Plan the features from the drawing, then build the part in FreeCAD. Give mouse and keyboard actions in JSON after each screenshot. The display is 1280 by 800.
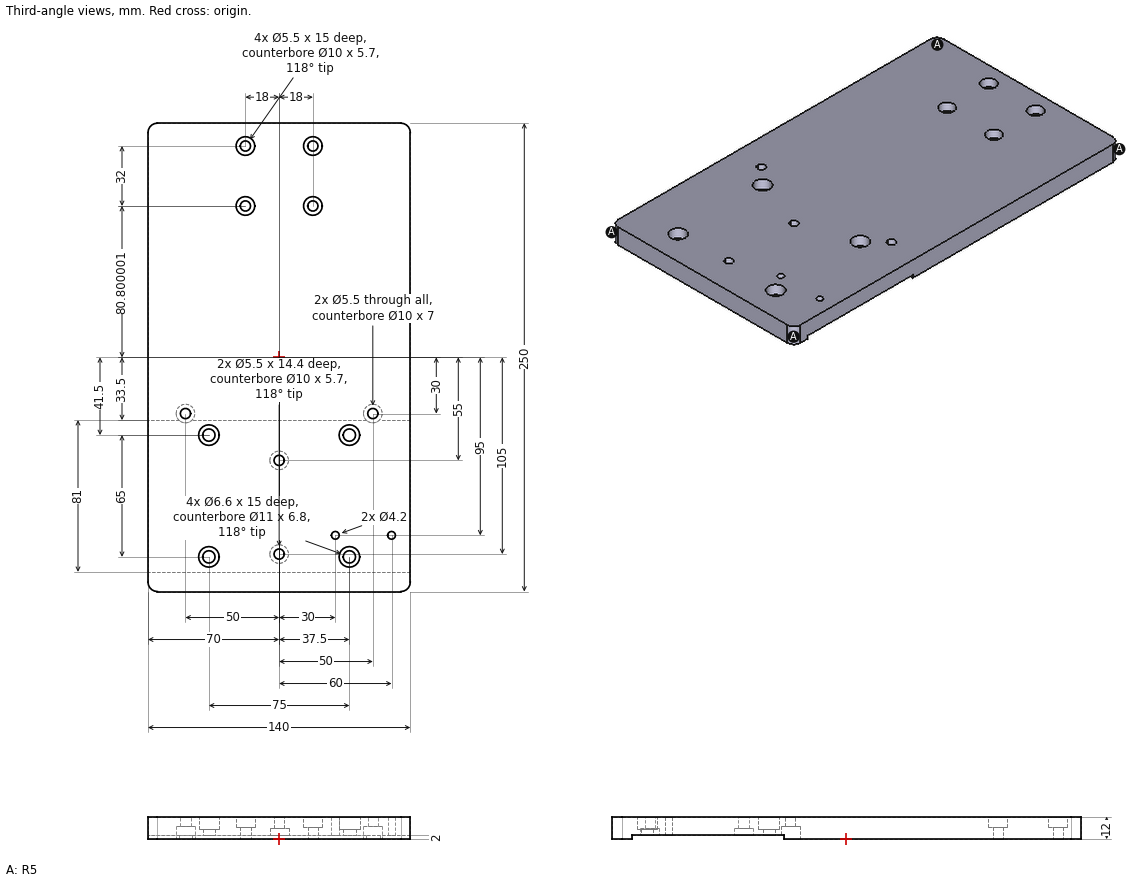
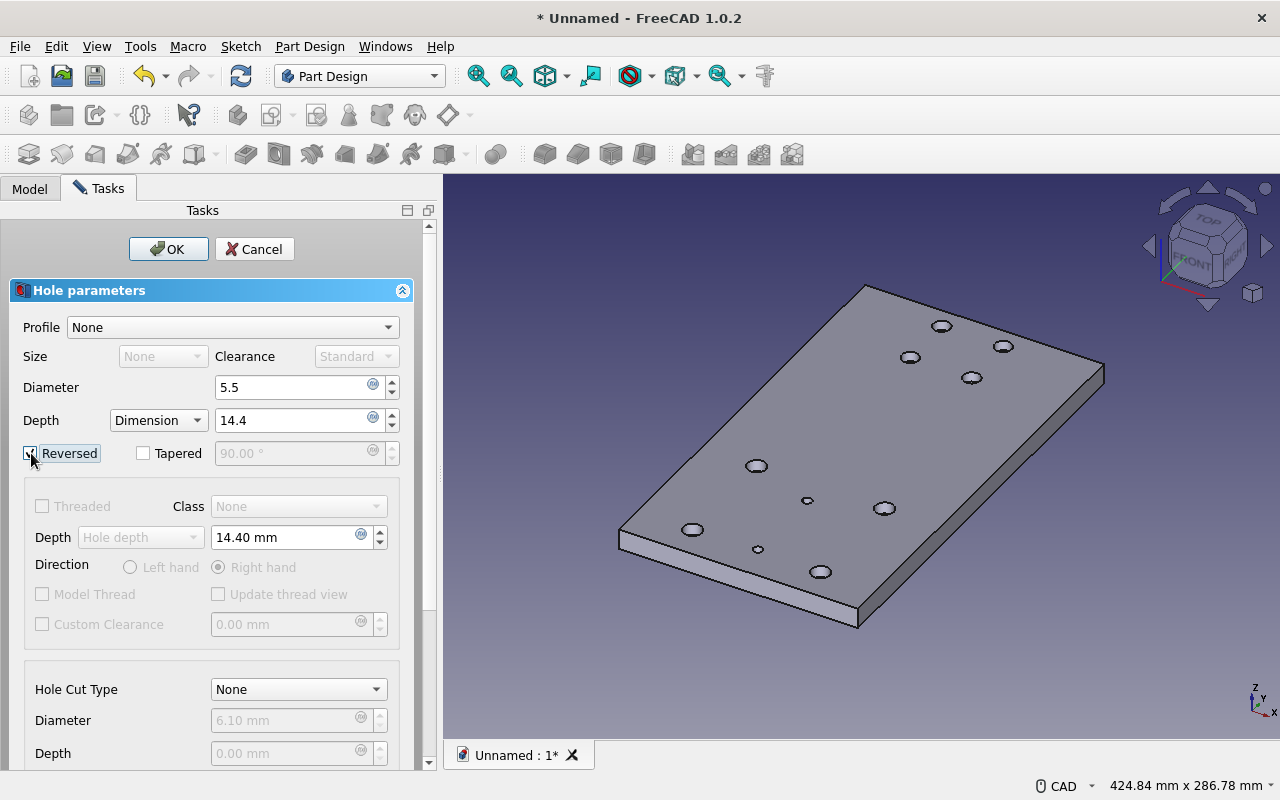
{"action": "left_click", "coordinate": [300, 690]}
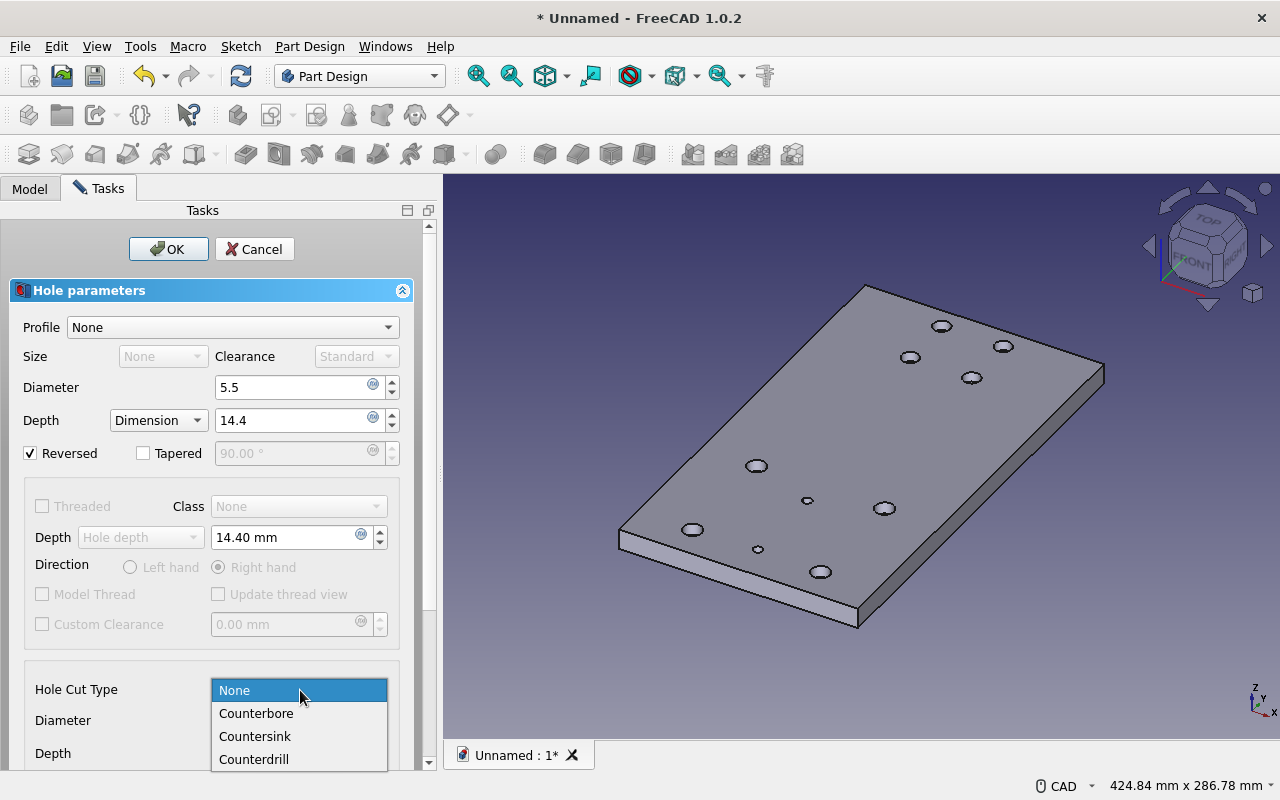
{"action": "left_click", "coordinate": [298, 714]}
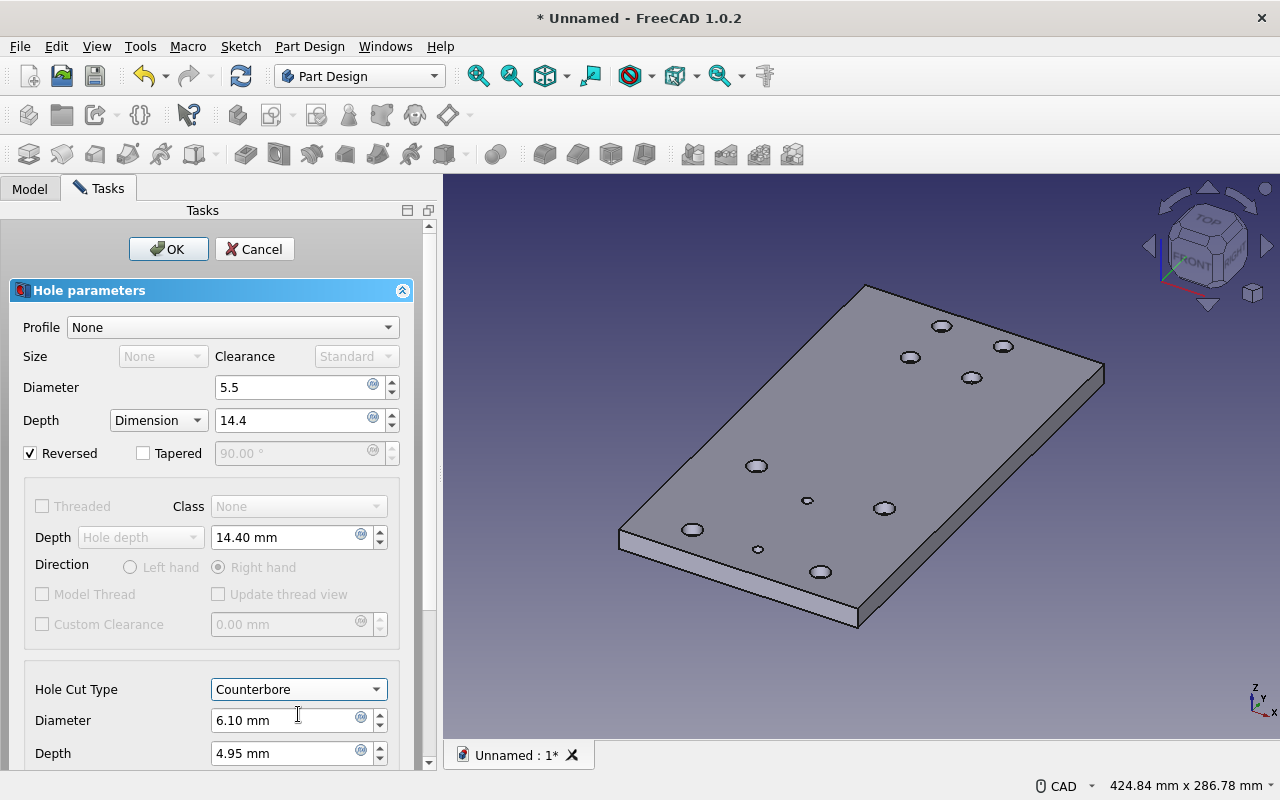
{"action": "triple_click", "coordinate": [292, 720]}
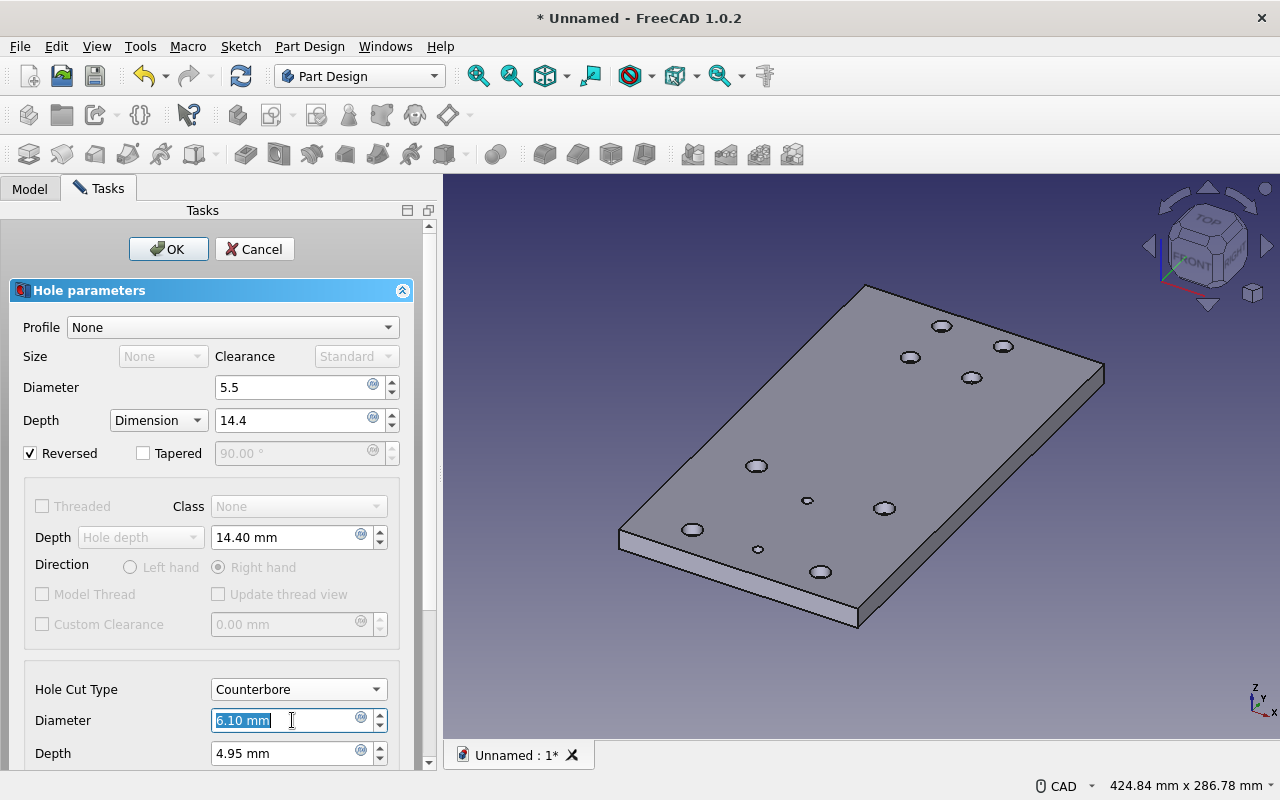
{"action": "type", "text": "10"}
{"action": "key", "text": "Tab"}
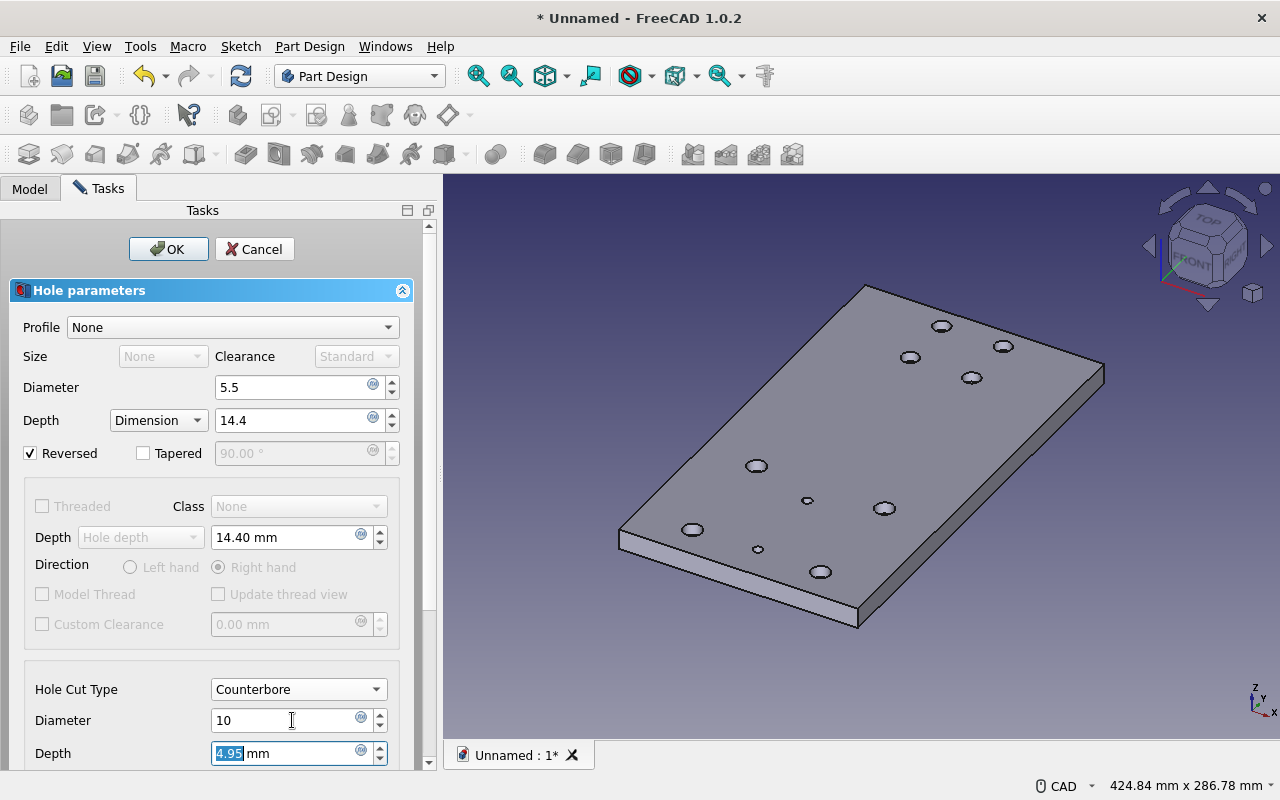
{"action": "type", "text": "5.7"}
{"action": "key", "text": "Tab"}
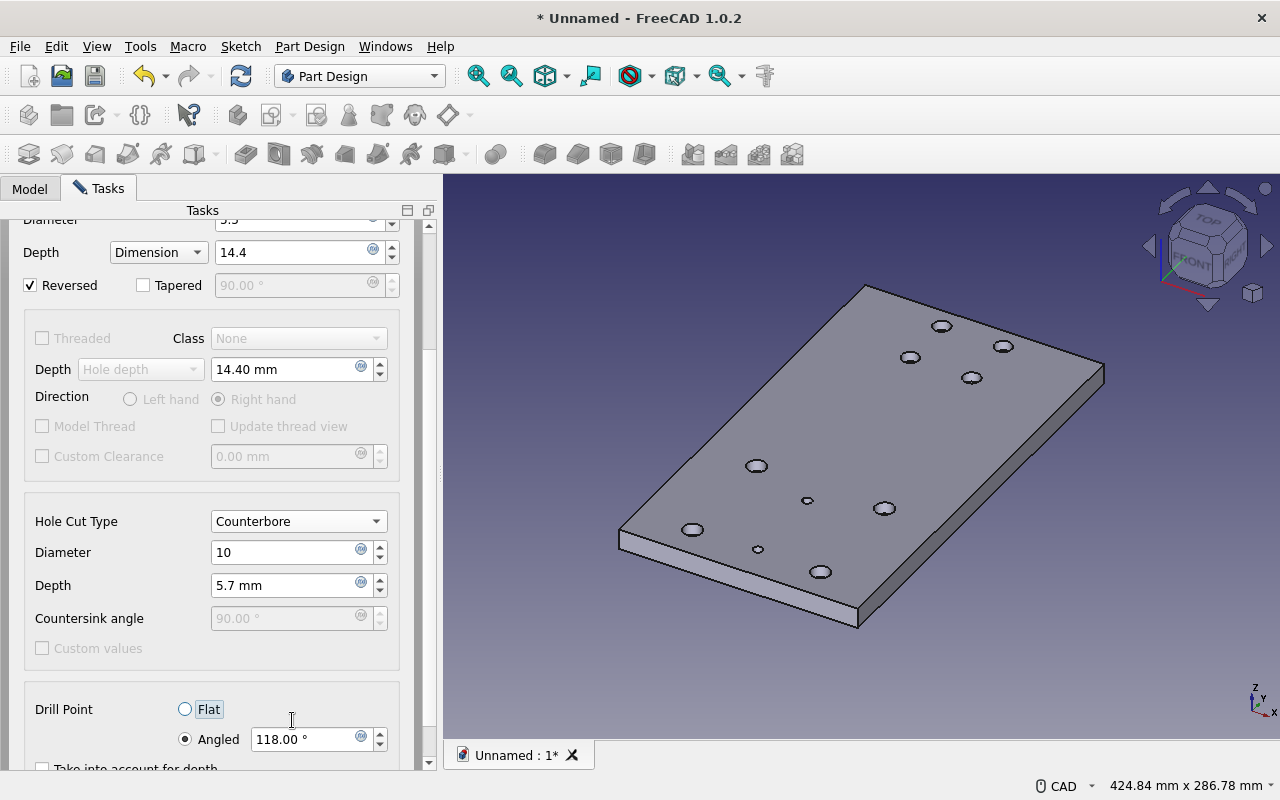
{"action": "scroll", "coordinate": [429, 495], "scroll_direction": "up", "scroll_amount": 4}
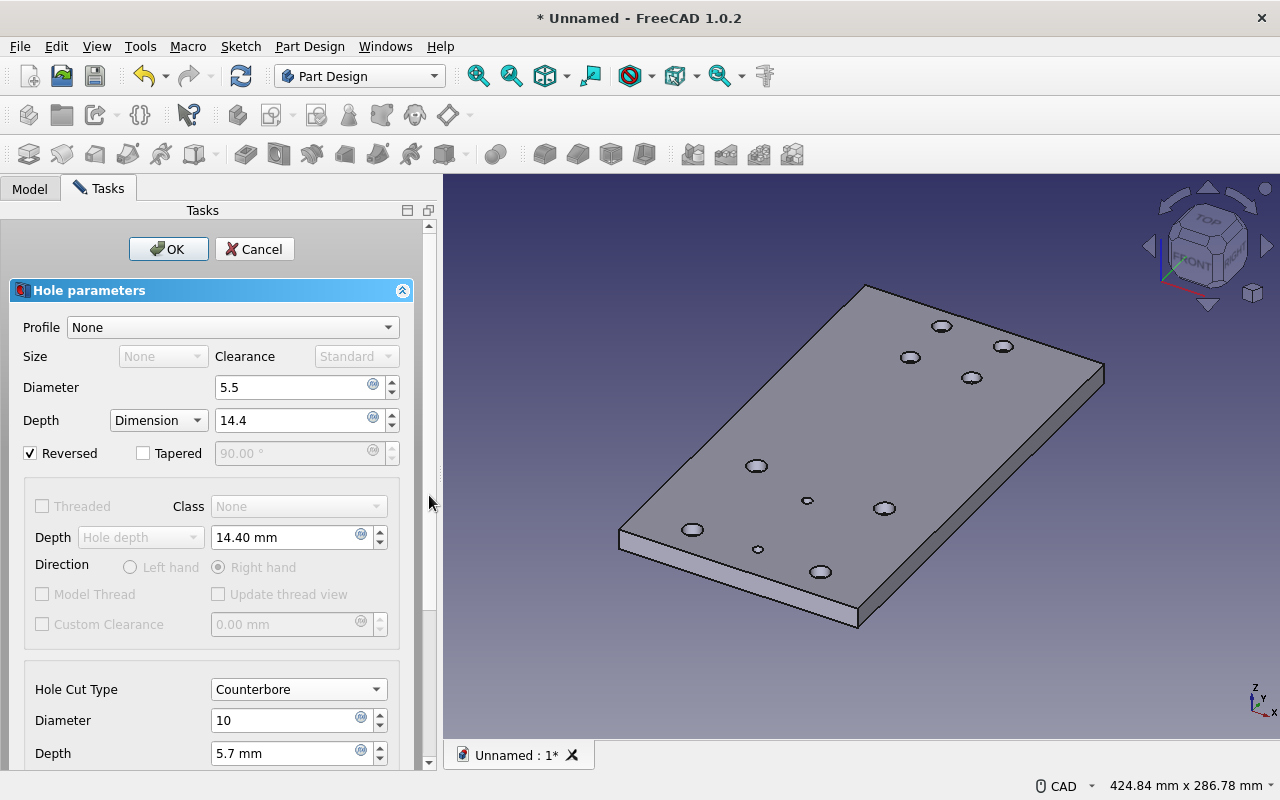
{"action": "left_click", "coordinate": [169, 249]}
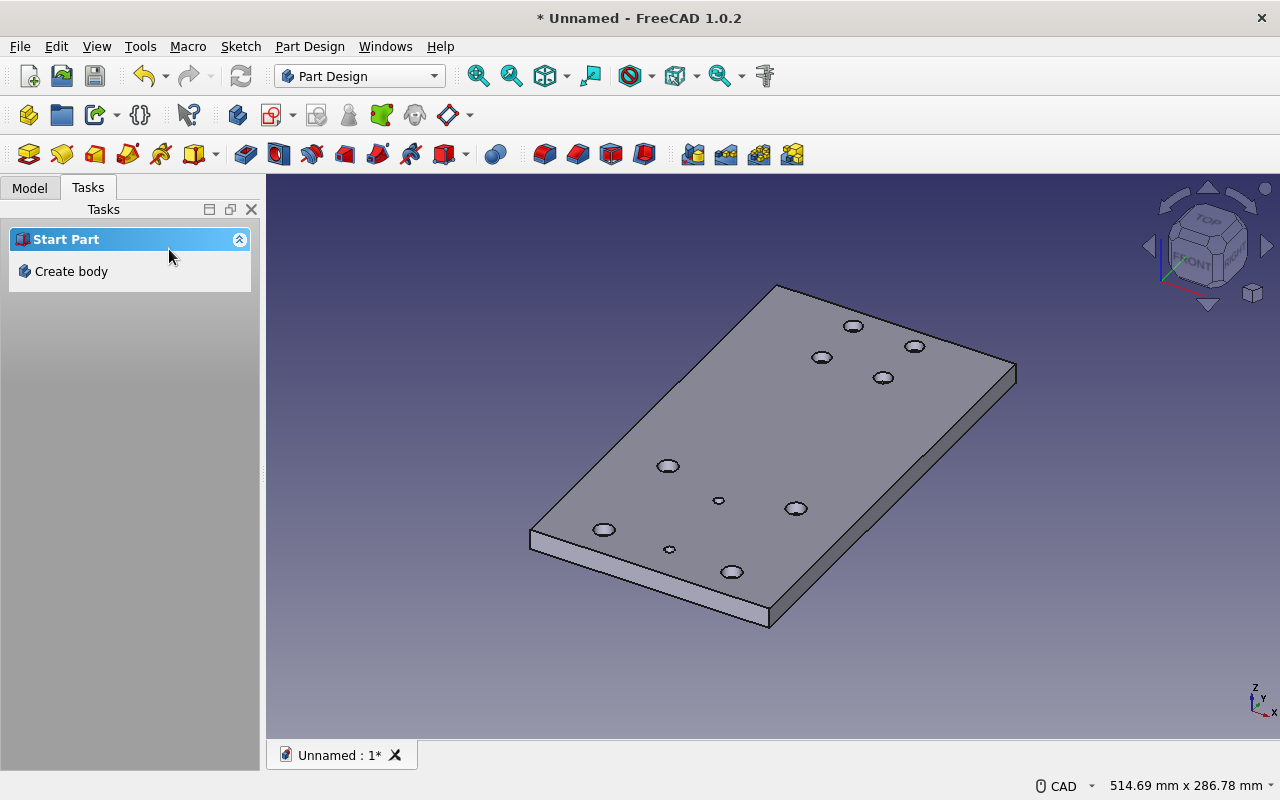
{"action": "left_click", "coordinate": [270, 116]}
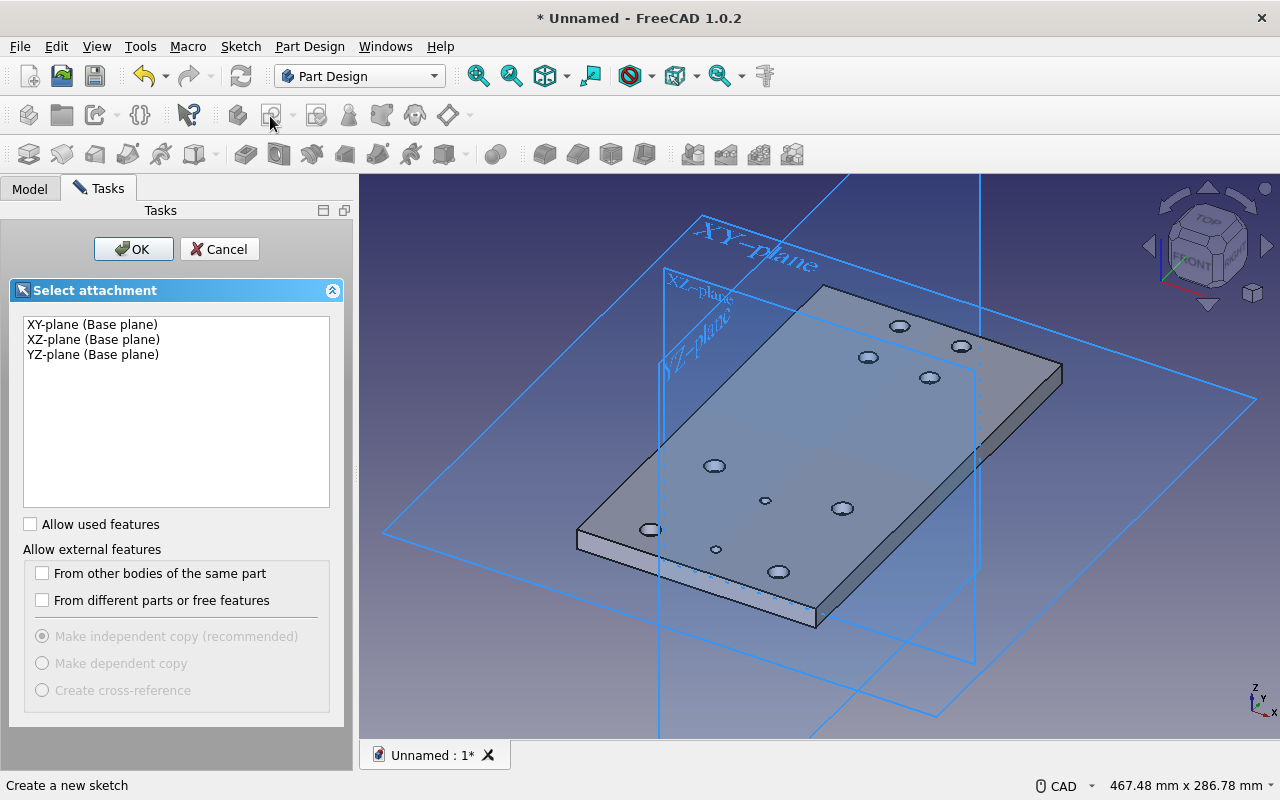
{"action": "left_click", "coordinate": [84, 324]}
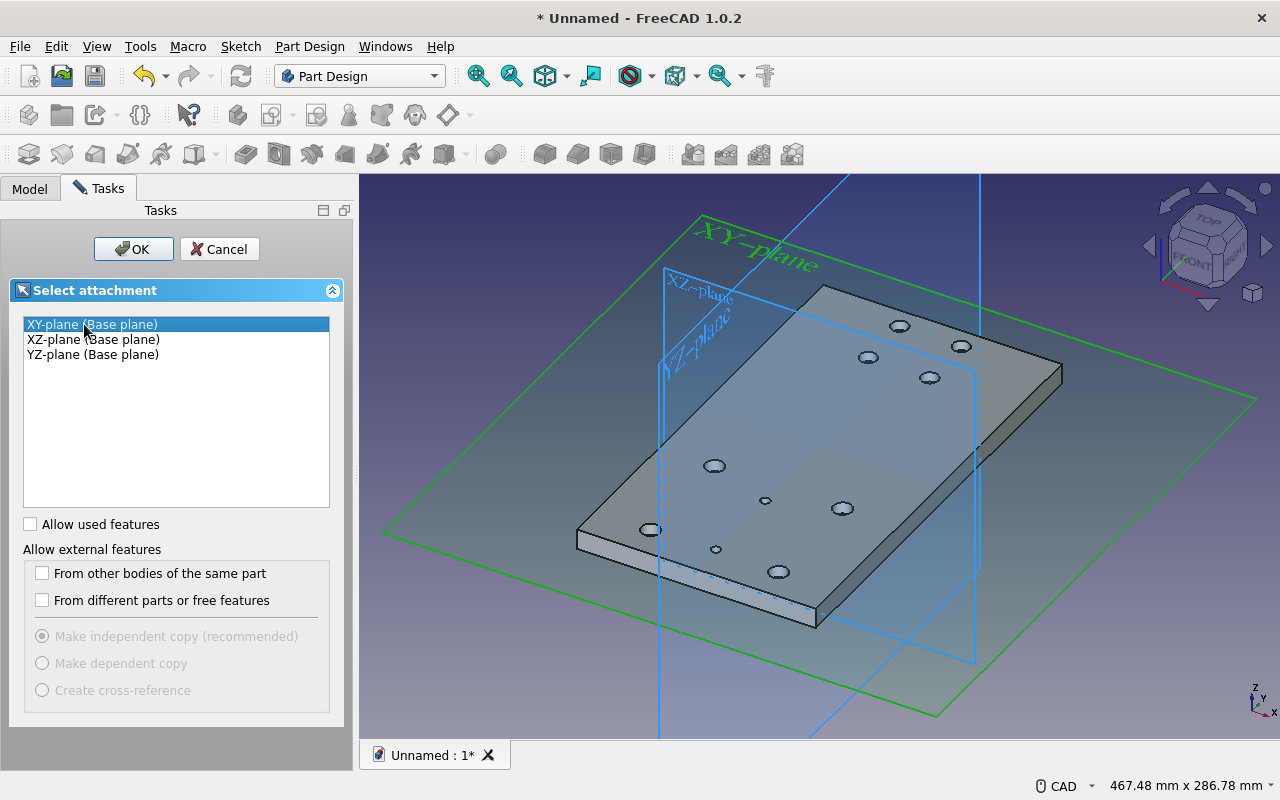
{"action": "left_click", "coordinate": [134, 249]}